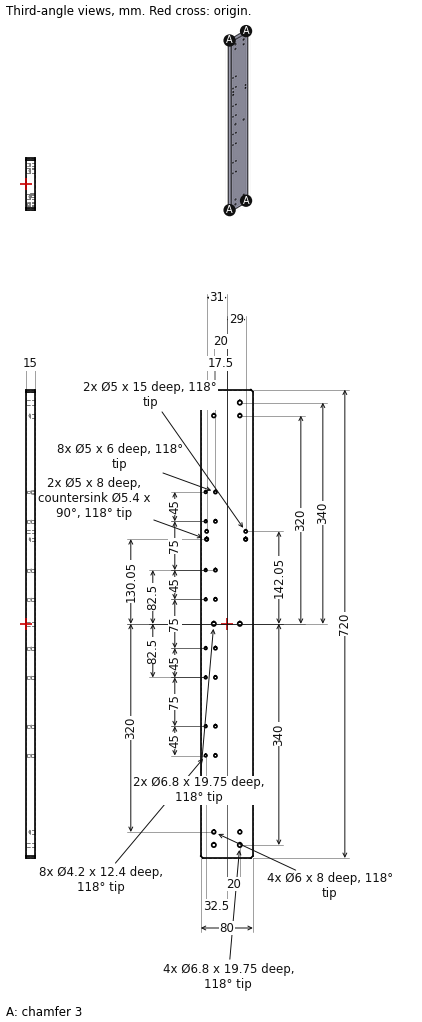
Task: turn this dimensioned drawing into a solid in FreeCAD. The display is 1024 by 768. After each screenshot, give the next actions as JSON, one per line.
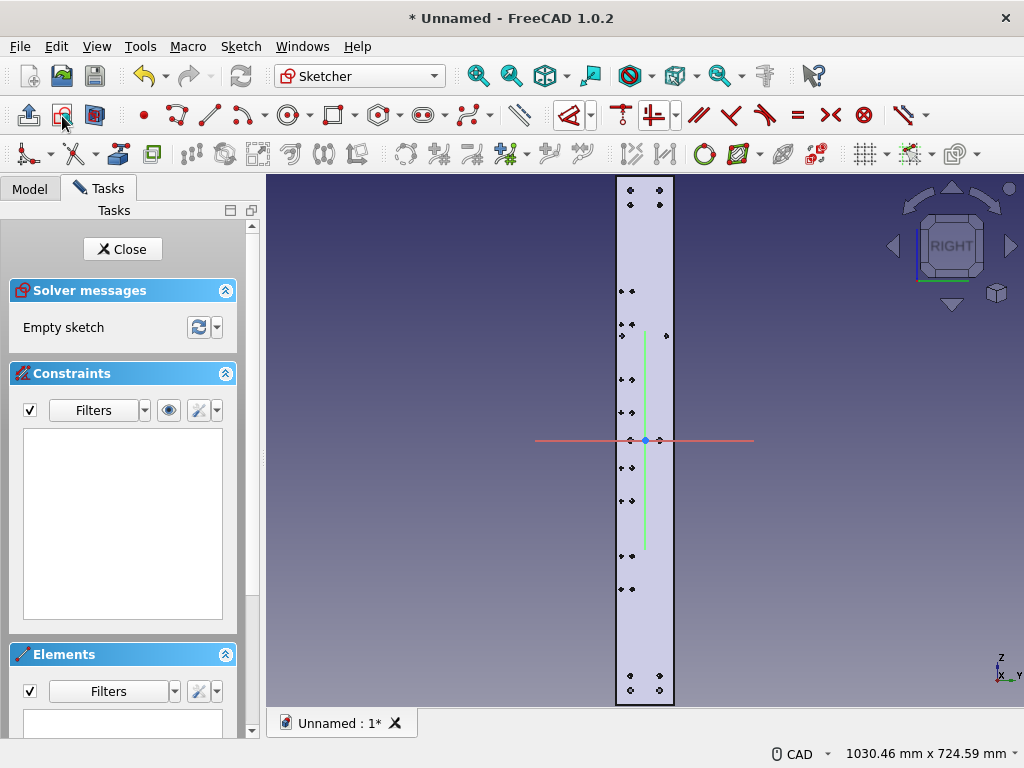
{"action": "scroll", "coordinate": [673, 371], "scroll_direction": "up", "scroll_amount": 6}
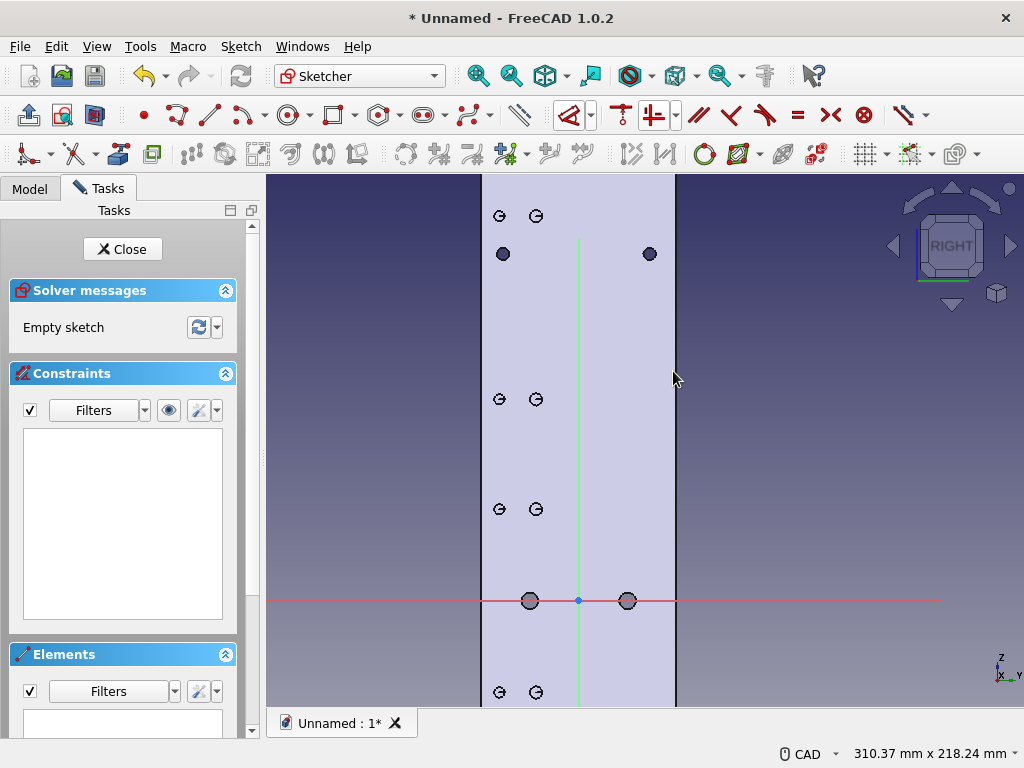
{"action": "key", "text": "g c"}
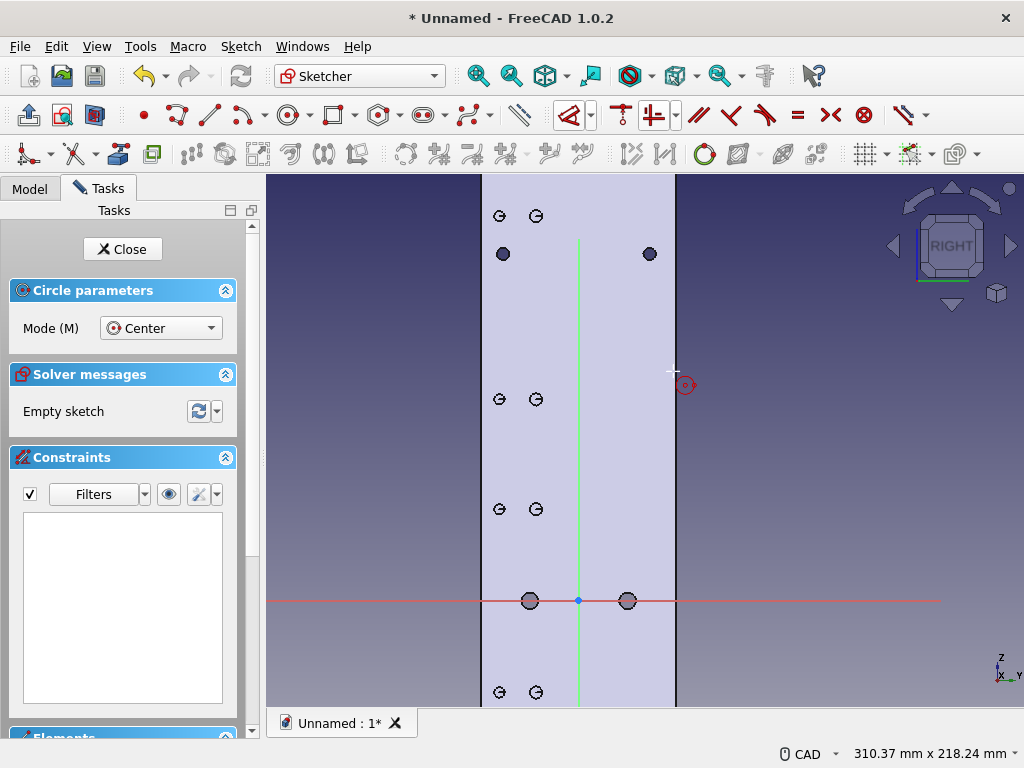
{"action": "scroll", "coordinate": [503, 283], "scroll_direction": "up", "scroll_amount": 7}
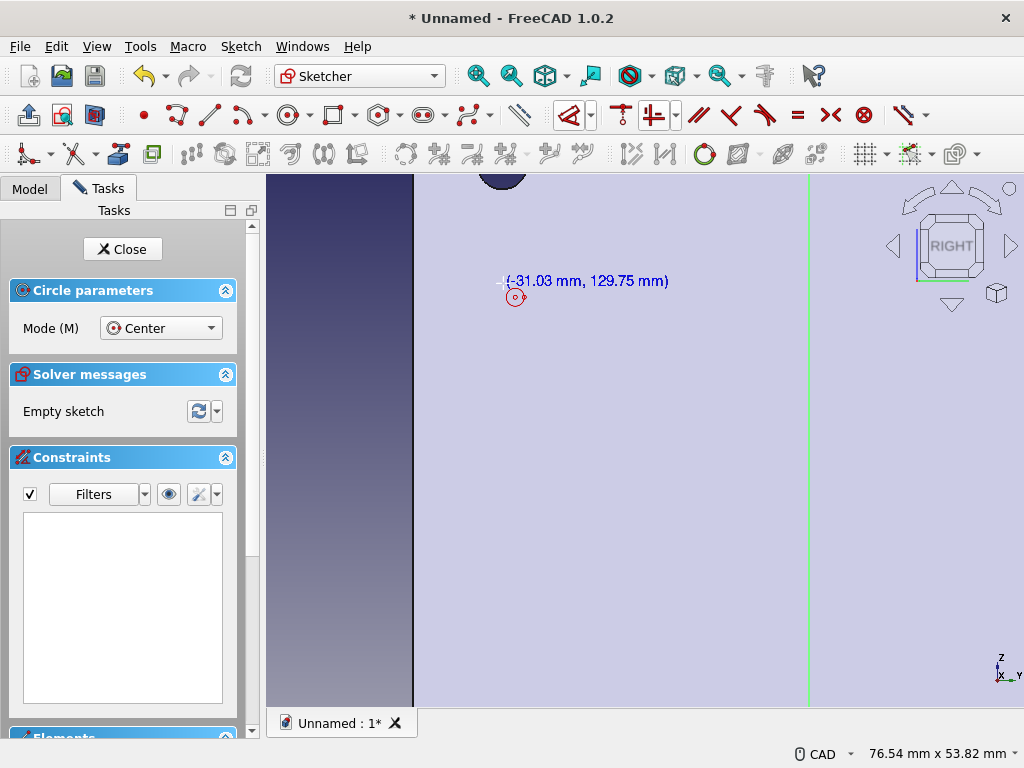
{"action": "scroll", "coordinate": [504, 285], "scroll_direction": "down", "scroll_amount": 7}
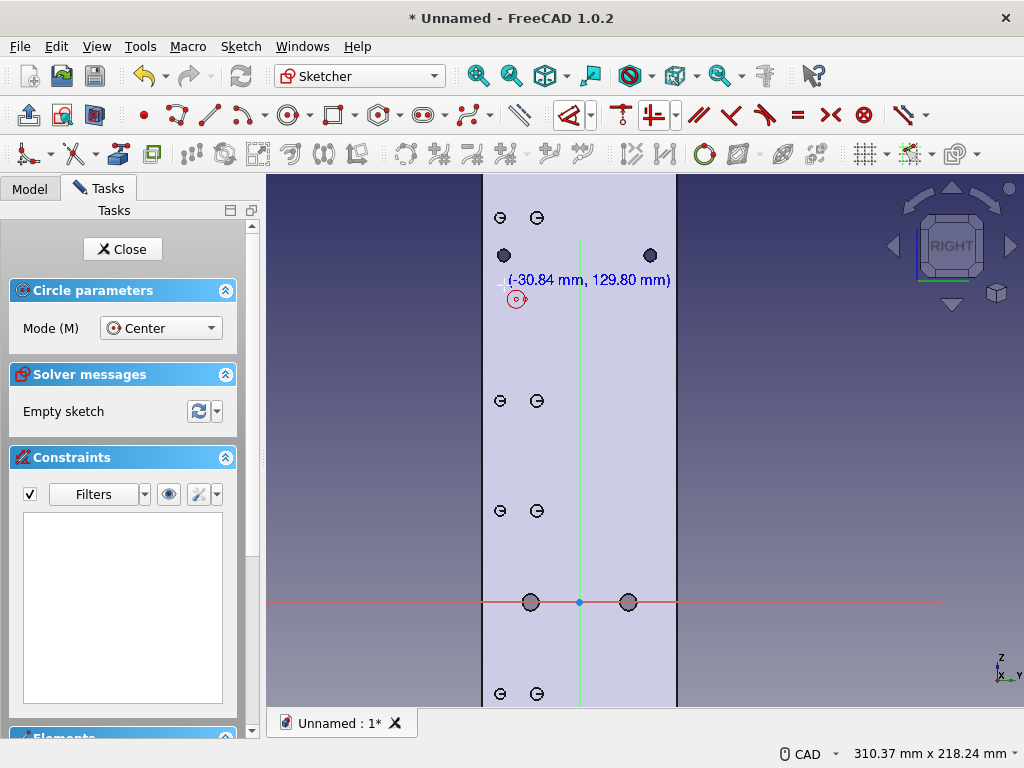
{"action": "left_click", "coordinate": [504, 285]}
{"action": "mouse_move", "coordinate": [508, 280]}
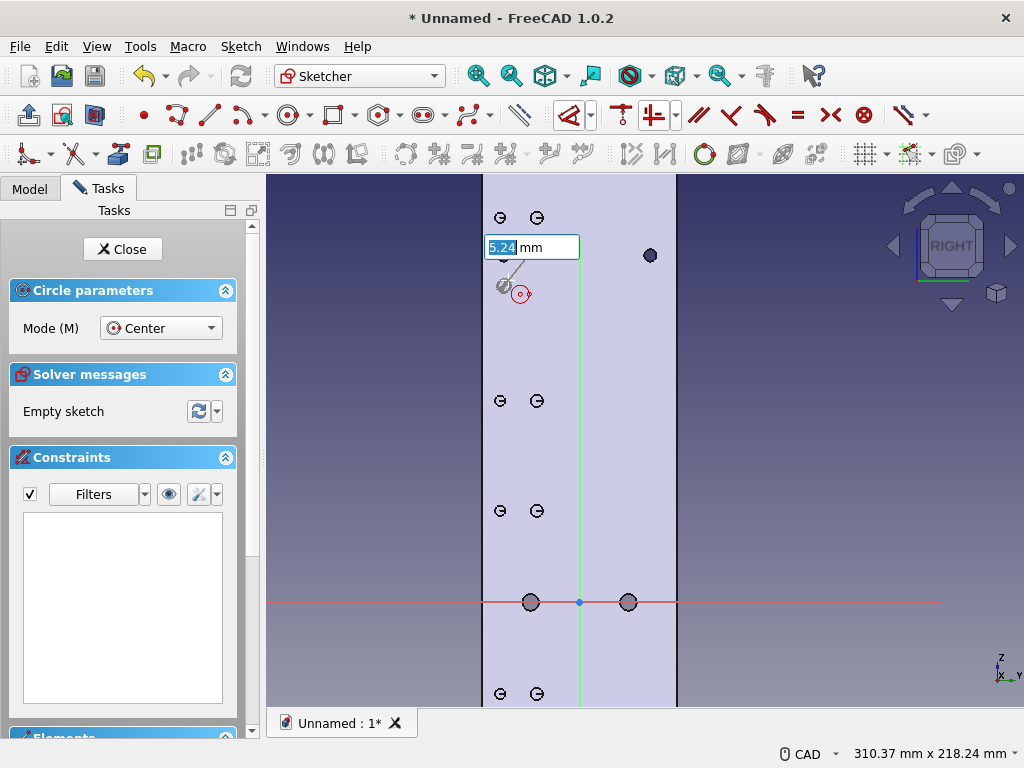
{"action": "type", "text": "5"}
{"action": "key", "text": "Return"}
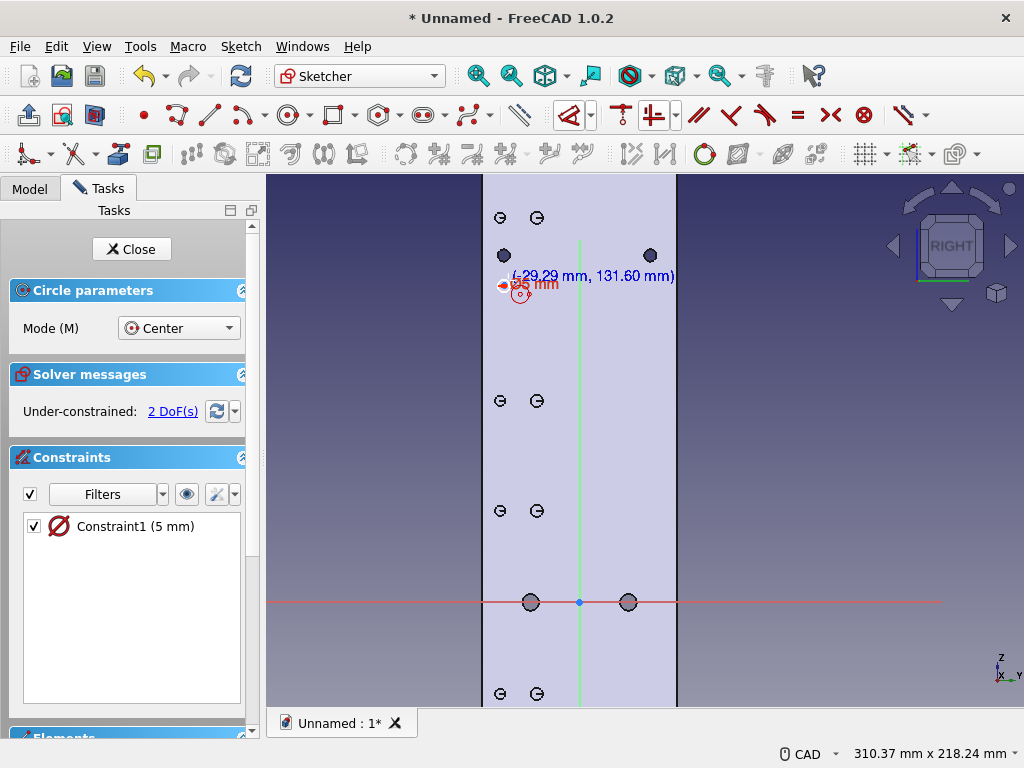
{"action": "scroll", "coordinate": [650, 285], "scroll_direction": "up", "scroll_amount": 7}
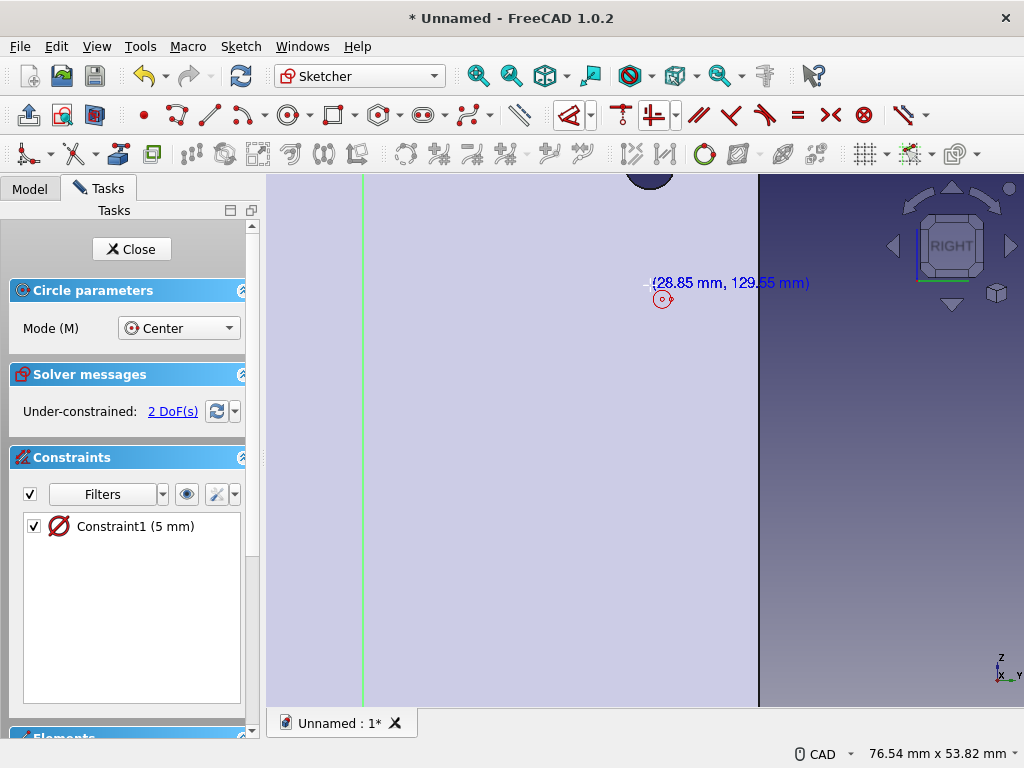
{"action": "scroll", "coordinate": [650, 285], "scroll_direction": "down", "scroll_amount": 7}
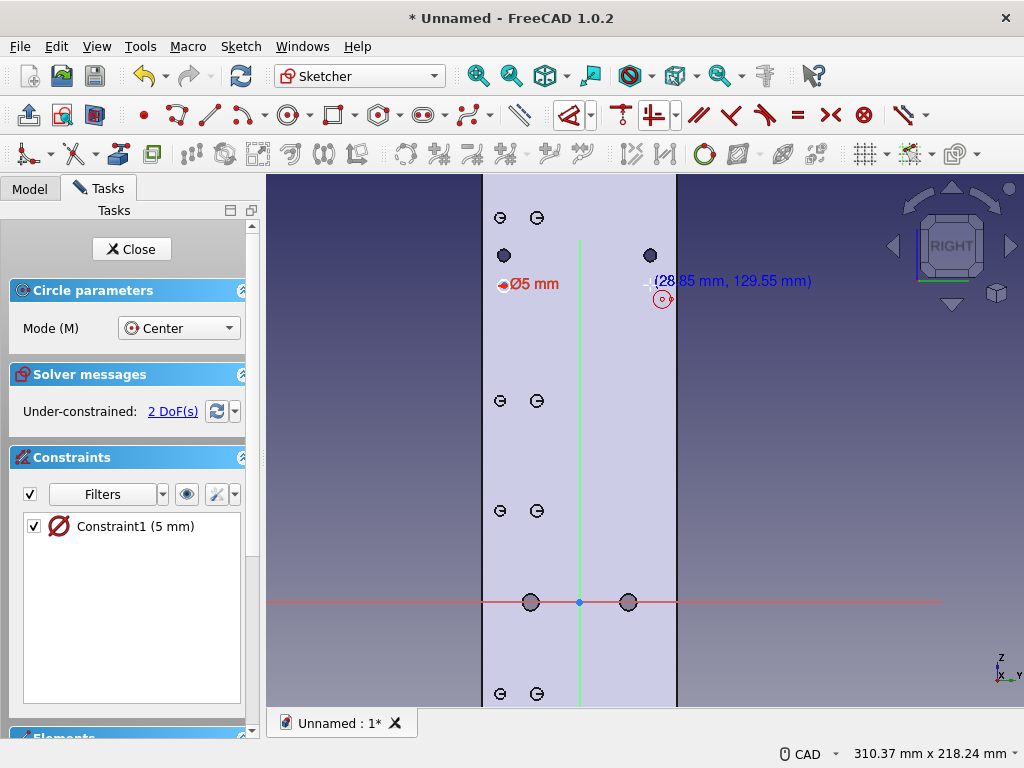
{"action": "left_click", "coordinate": [650, 285]}
{"action": "mouse_move", "coordinate": [655, 280]}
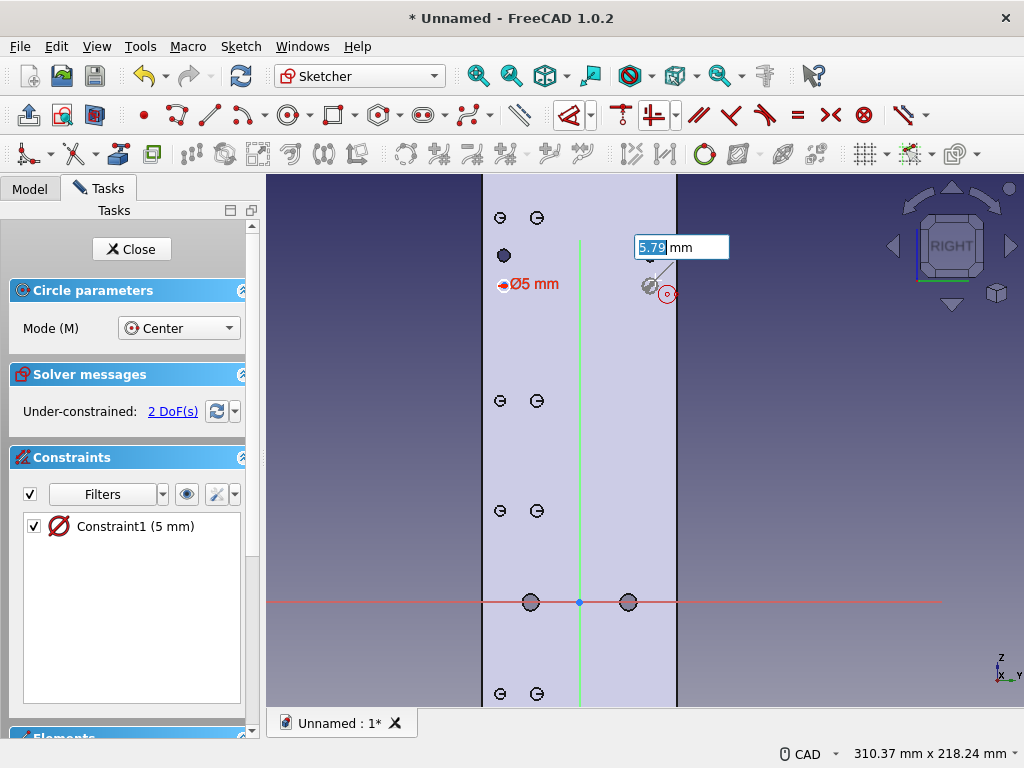
{"action": "type", "text": "5"}
{"action": "key", "text": "Return"}
{"action": "key", "text": "Escape"}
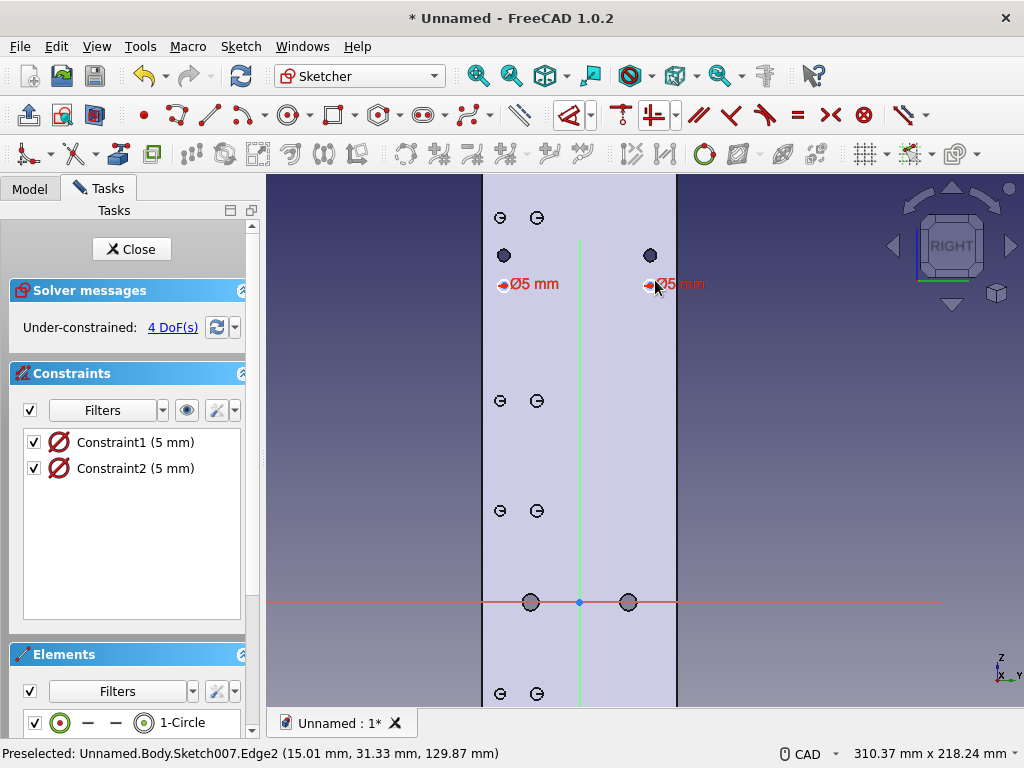
{"action": "left_click", "coordinate": [504, 286]}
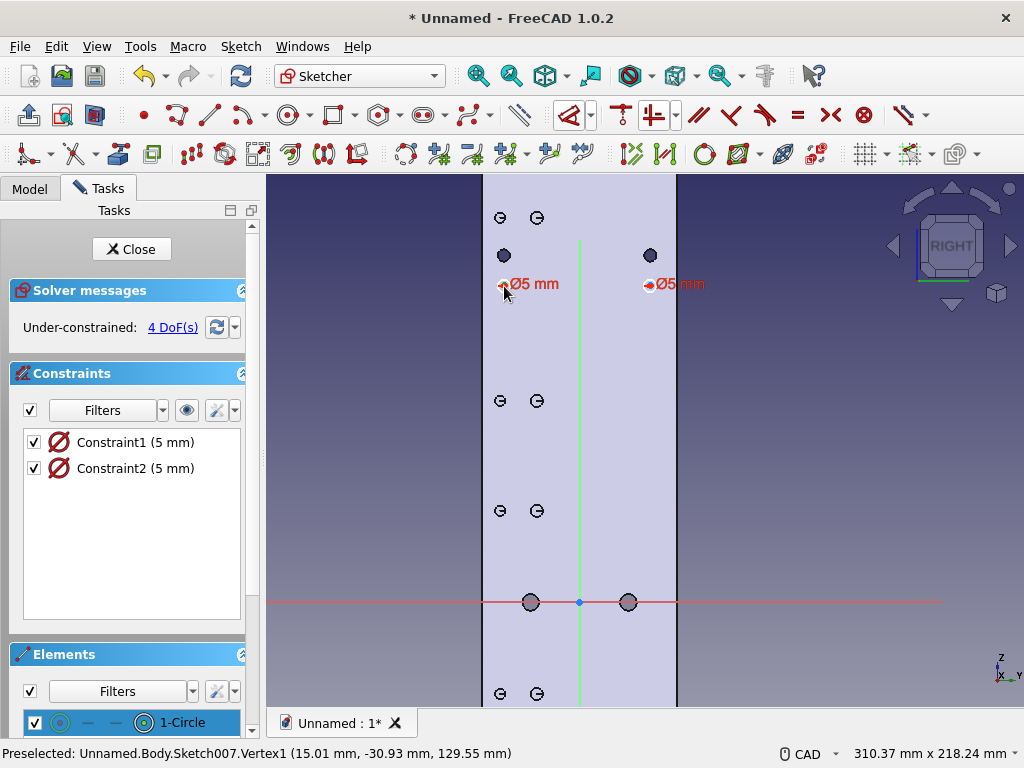
{"action": "left_click", "coordinate": [650, 286]}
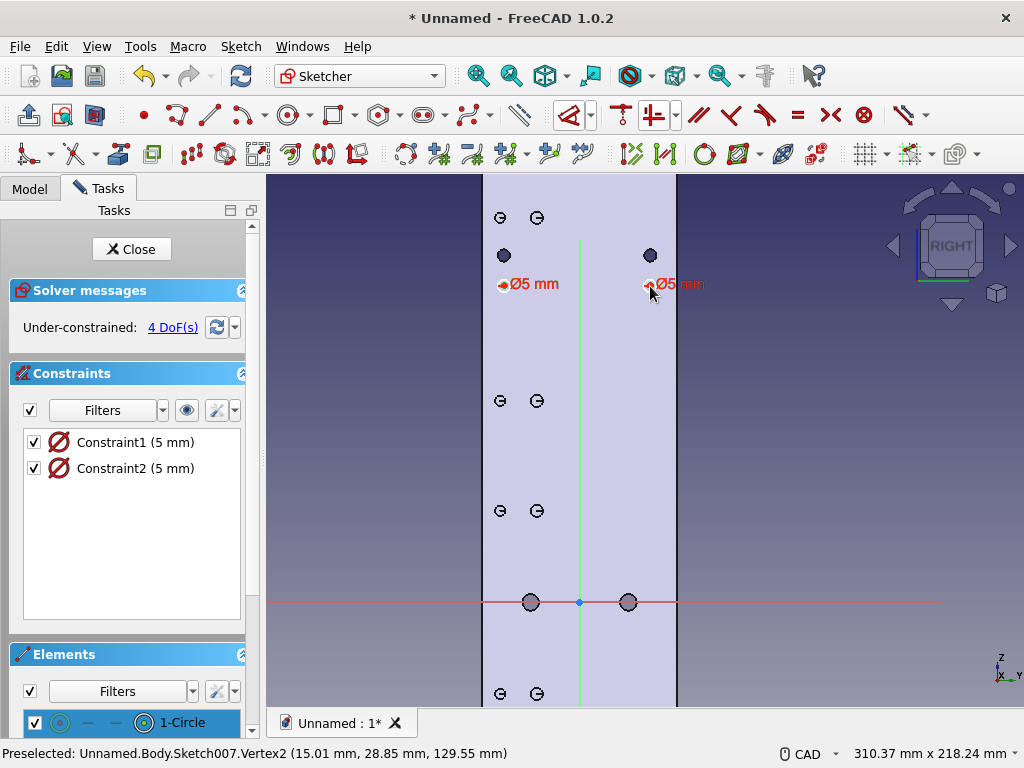
{"action": "left_click", "coordinate": [676, 116]}